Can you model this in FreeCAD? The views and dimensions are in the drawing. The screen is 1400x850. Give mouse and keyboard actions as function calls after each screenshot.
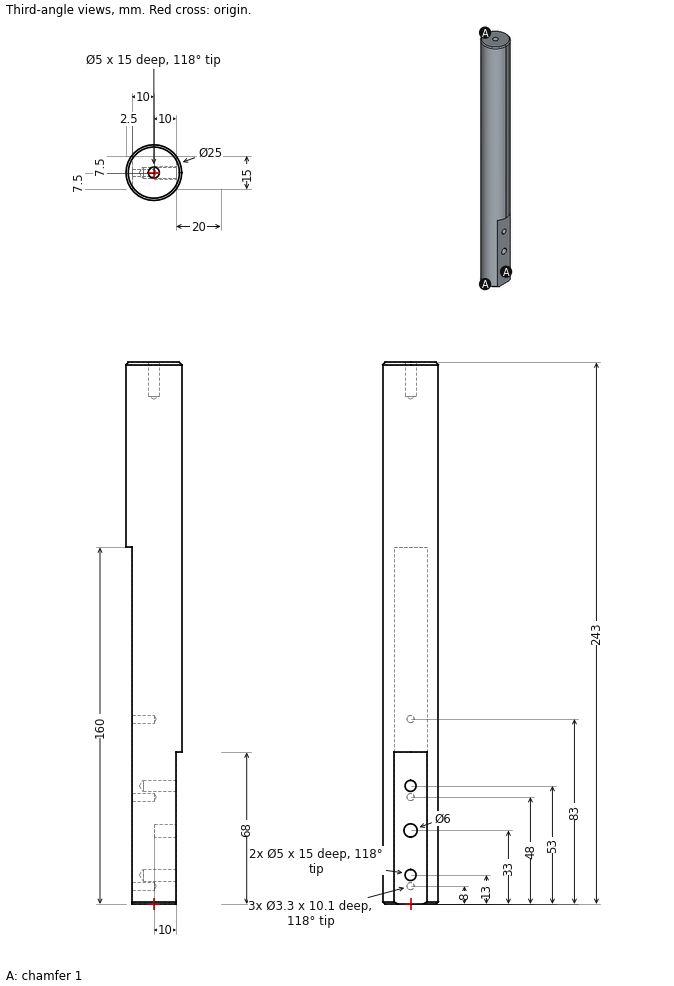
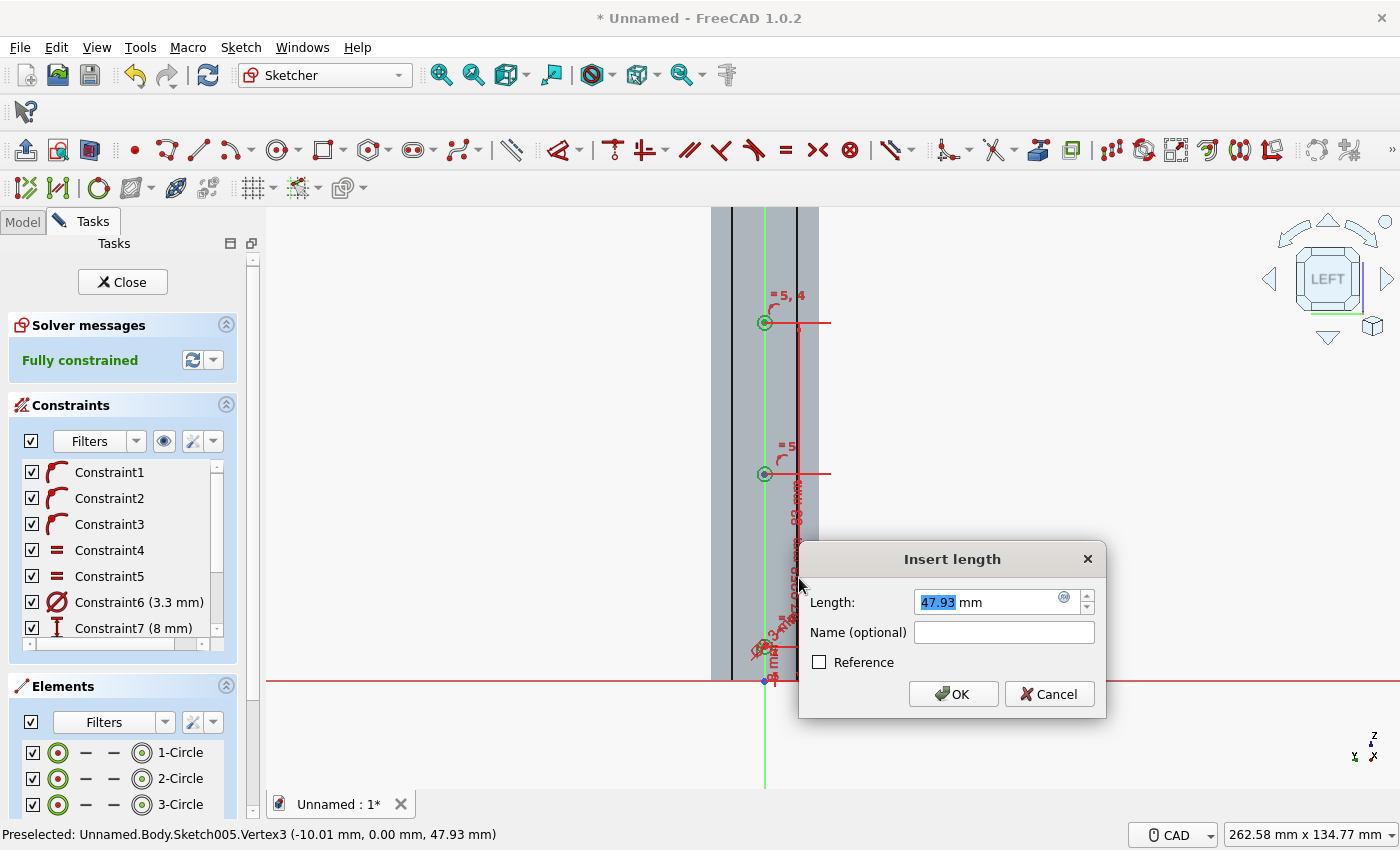
text(48)
key(Return)
key(Escape)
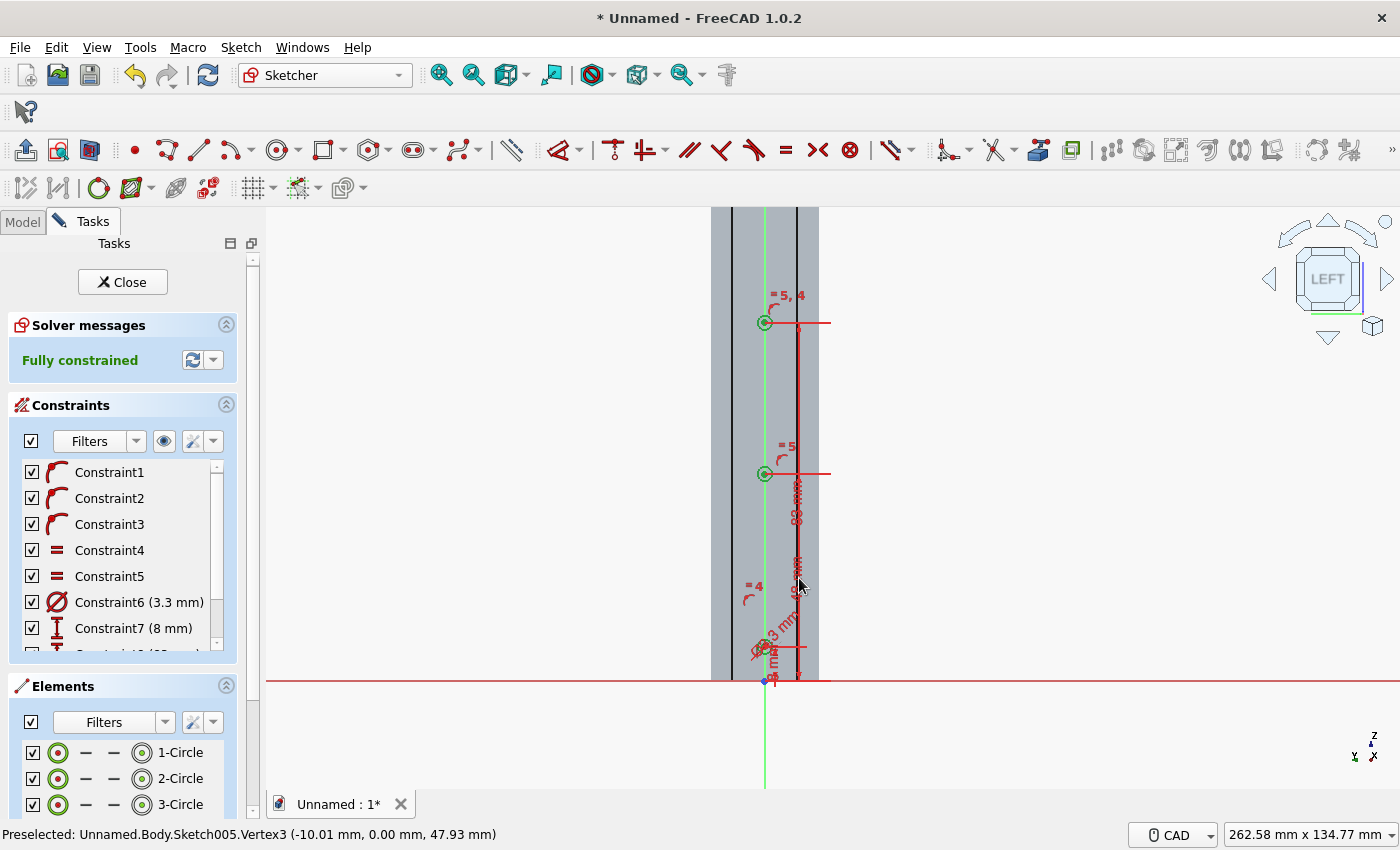
click(123, 282)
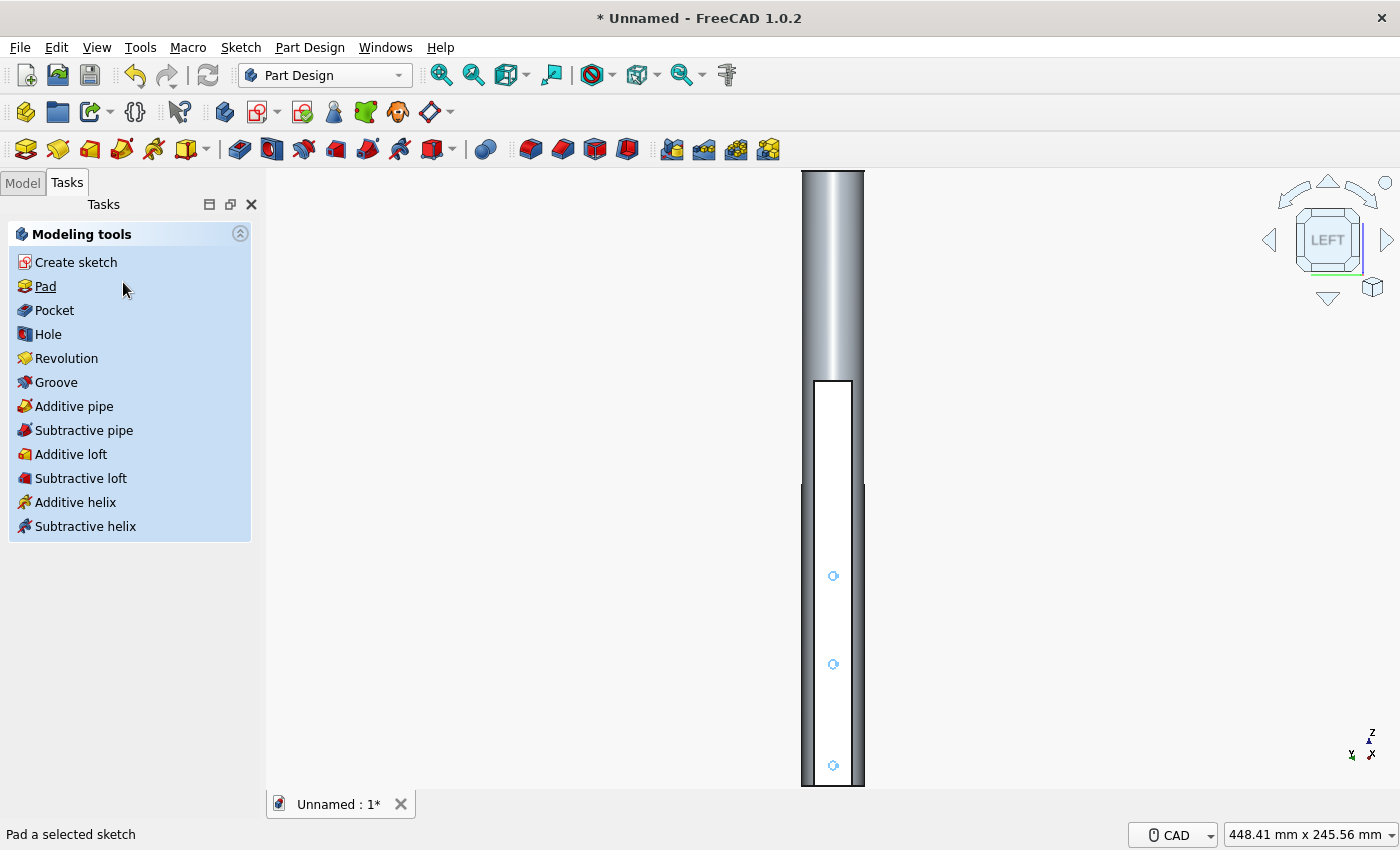
click(272, 150)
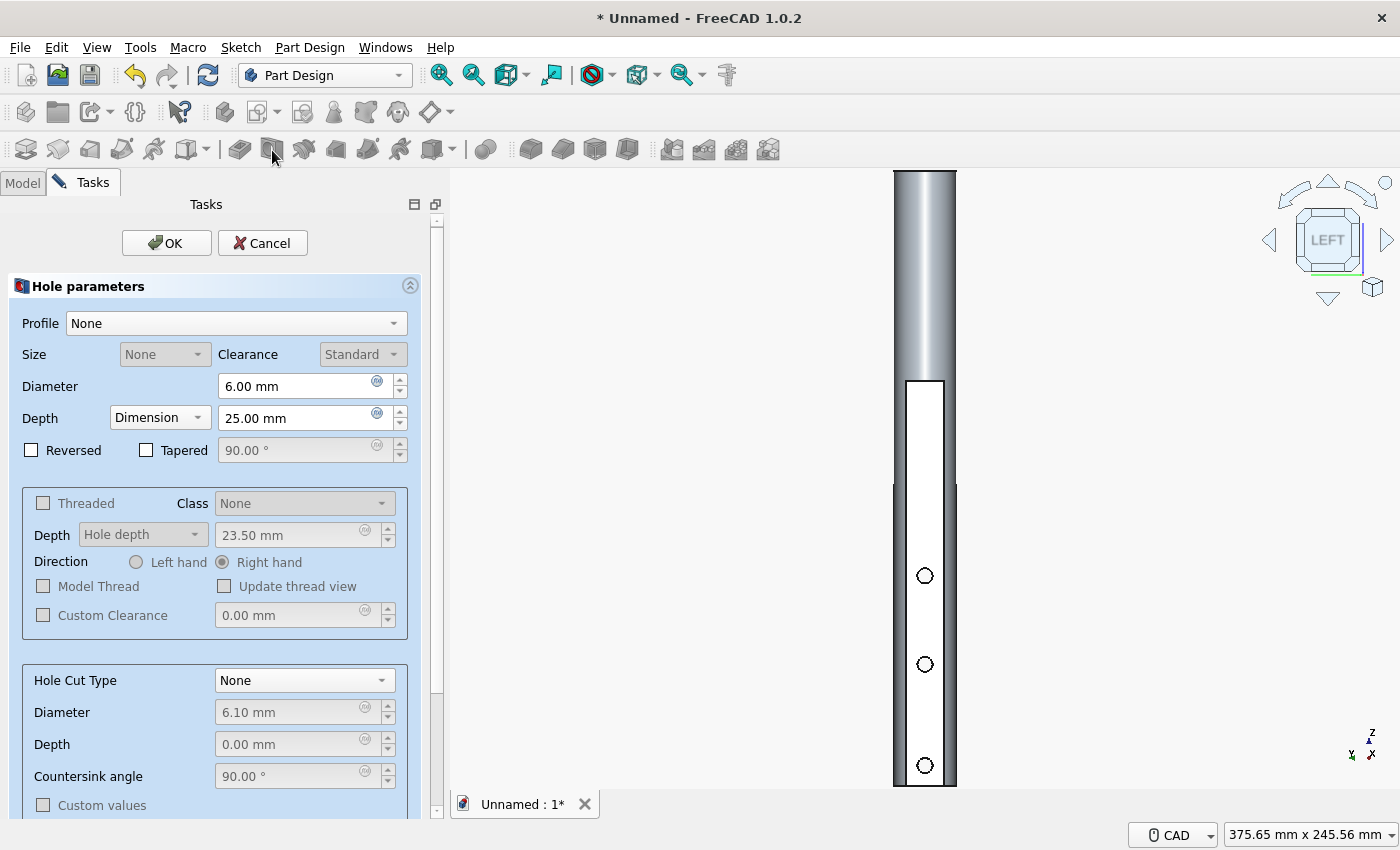
triple_click(305, 386)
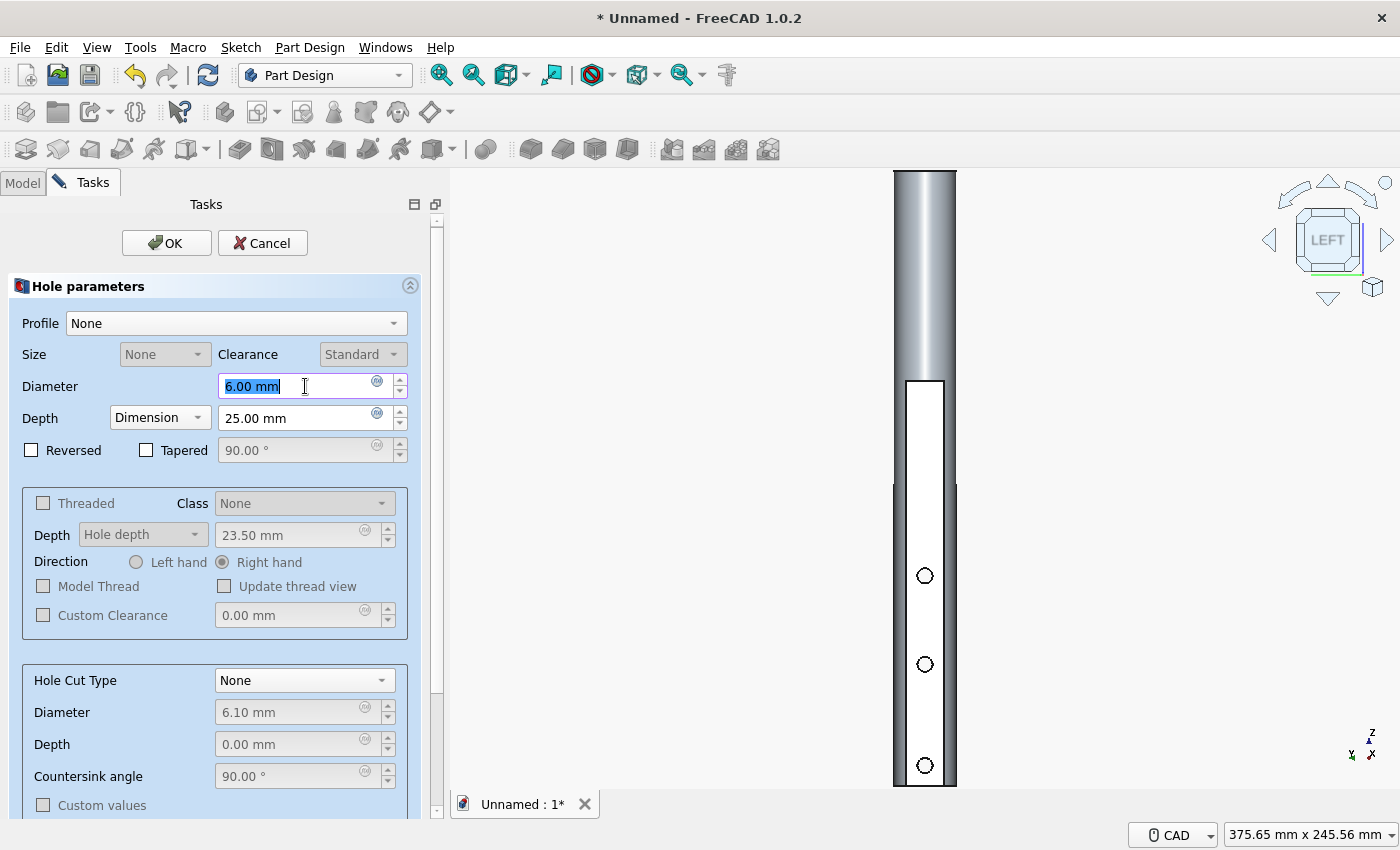
text(3.3)
key(Tab)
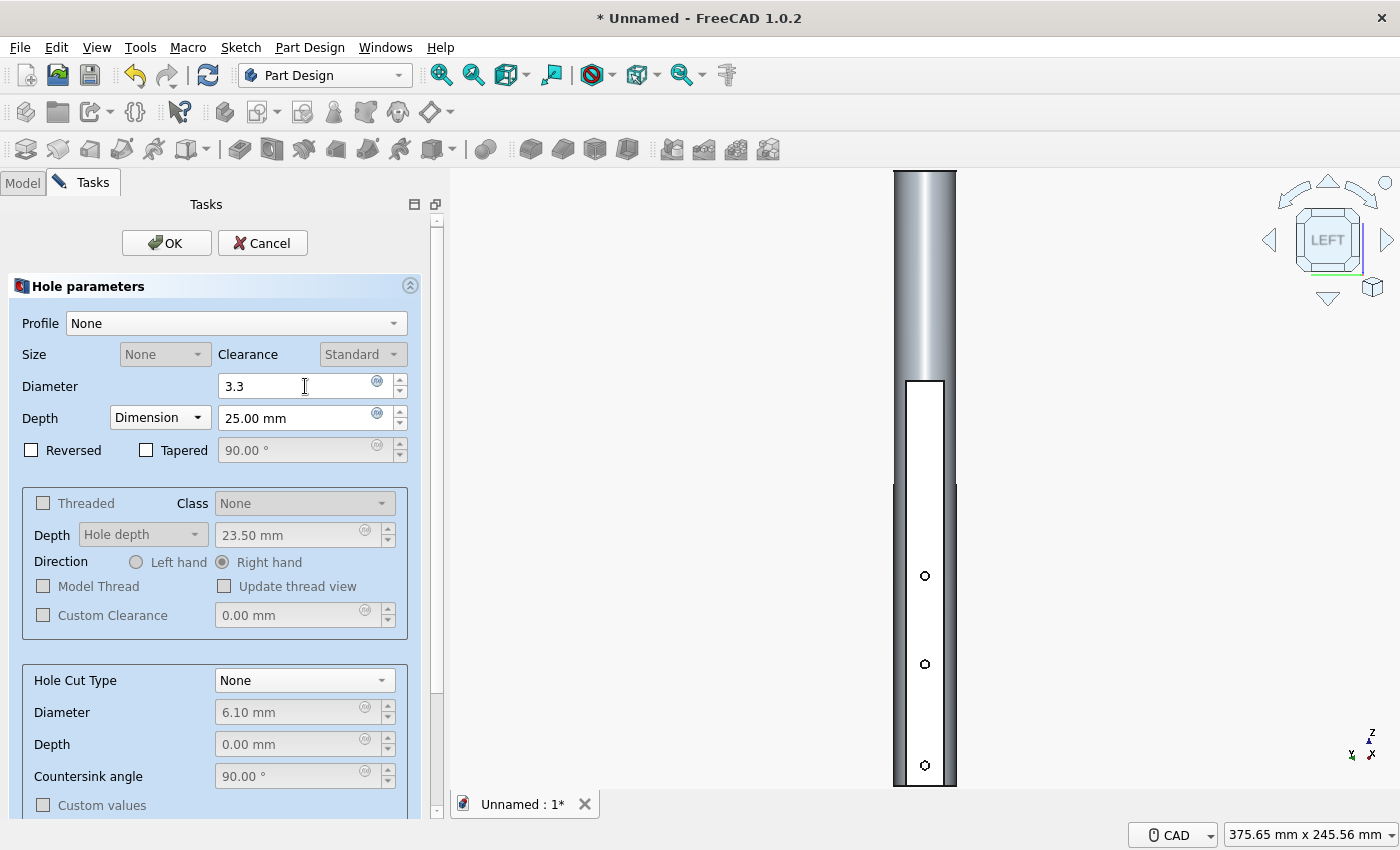
triple_click(305, 418)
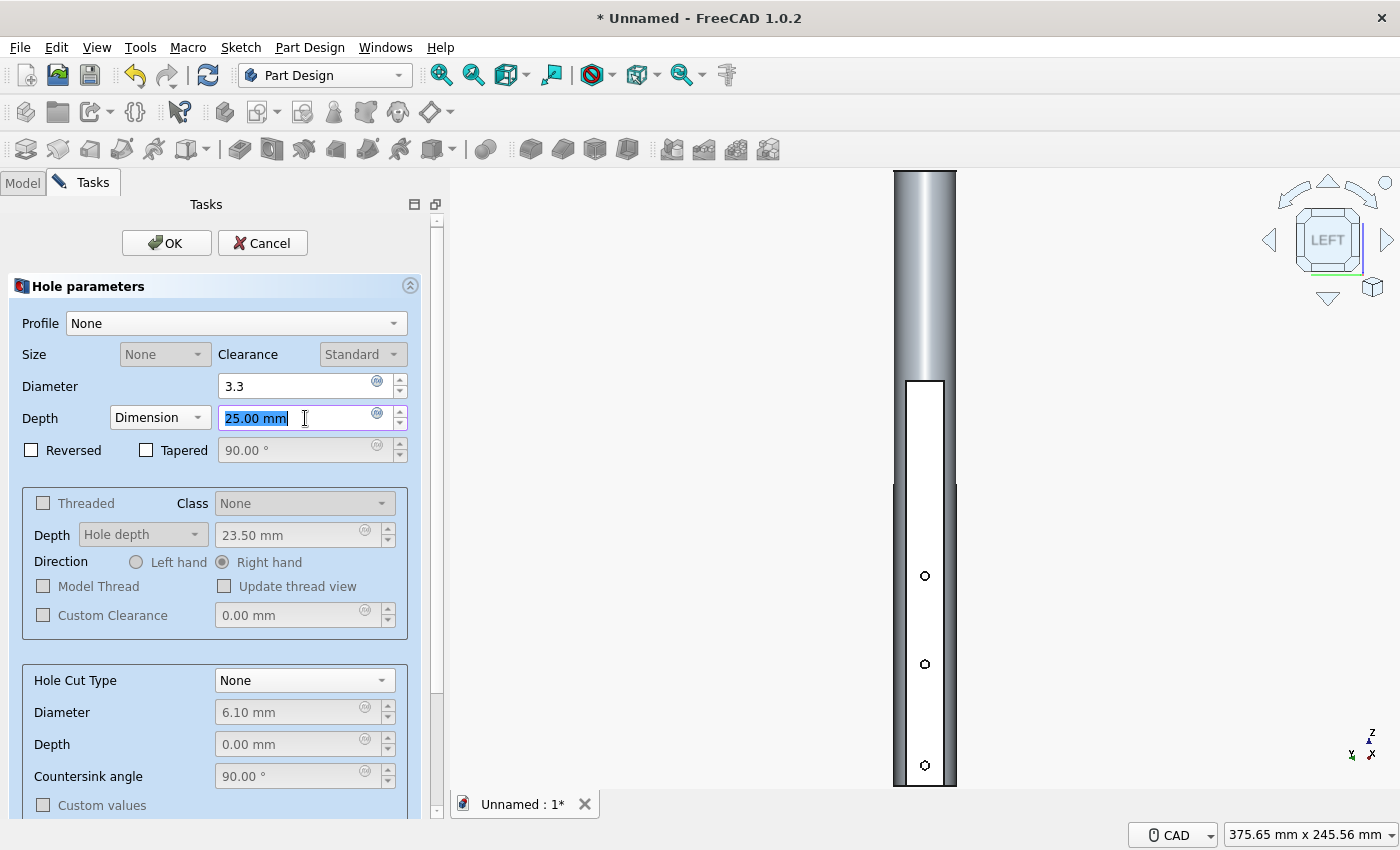
text(10.1)
key(Tab)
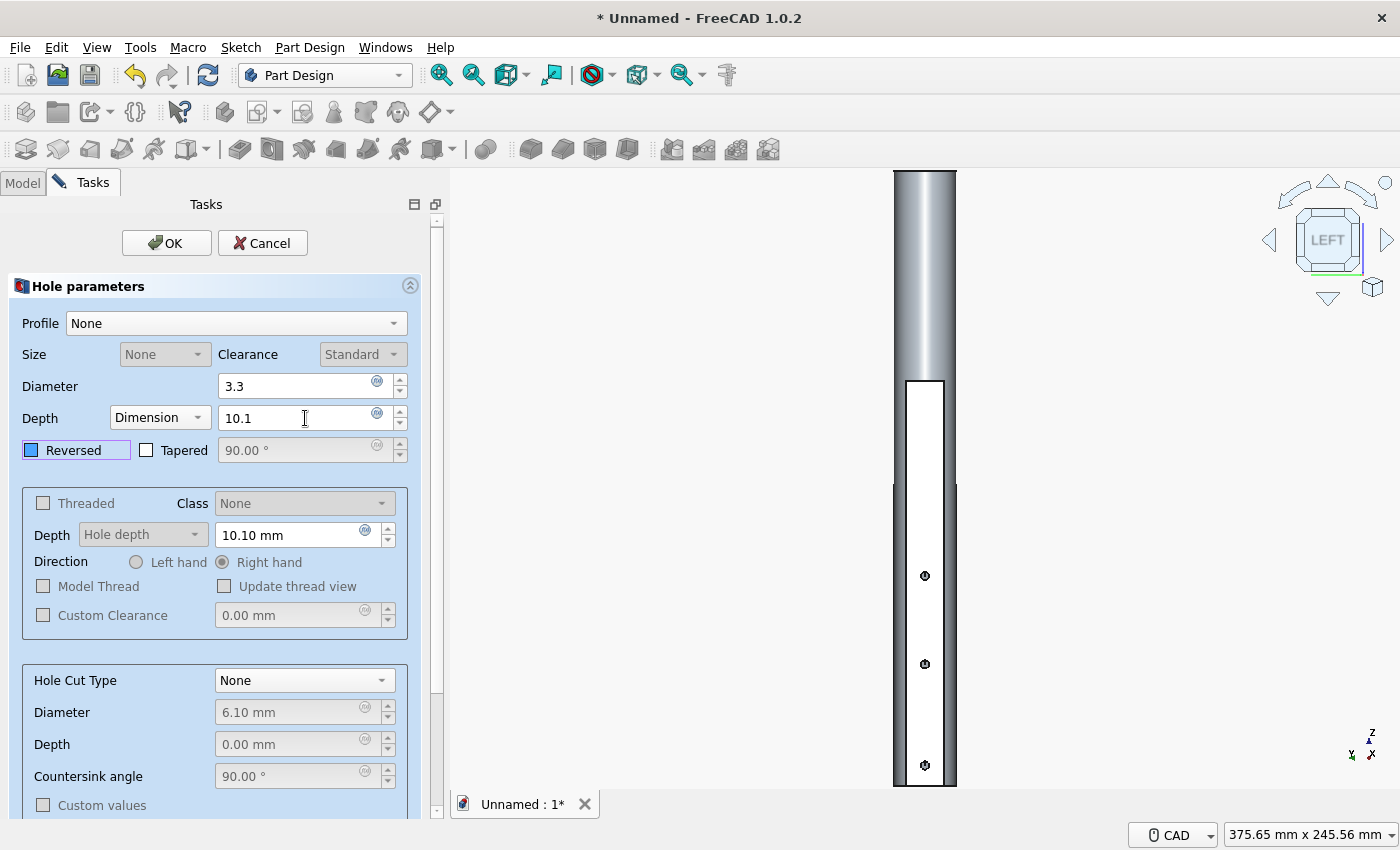
click(167, 243)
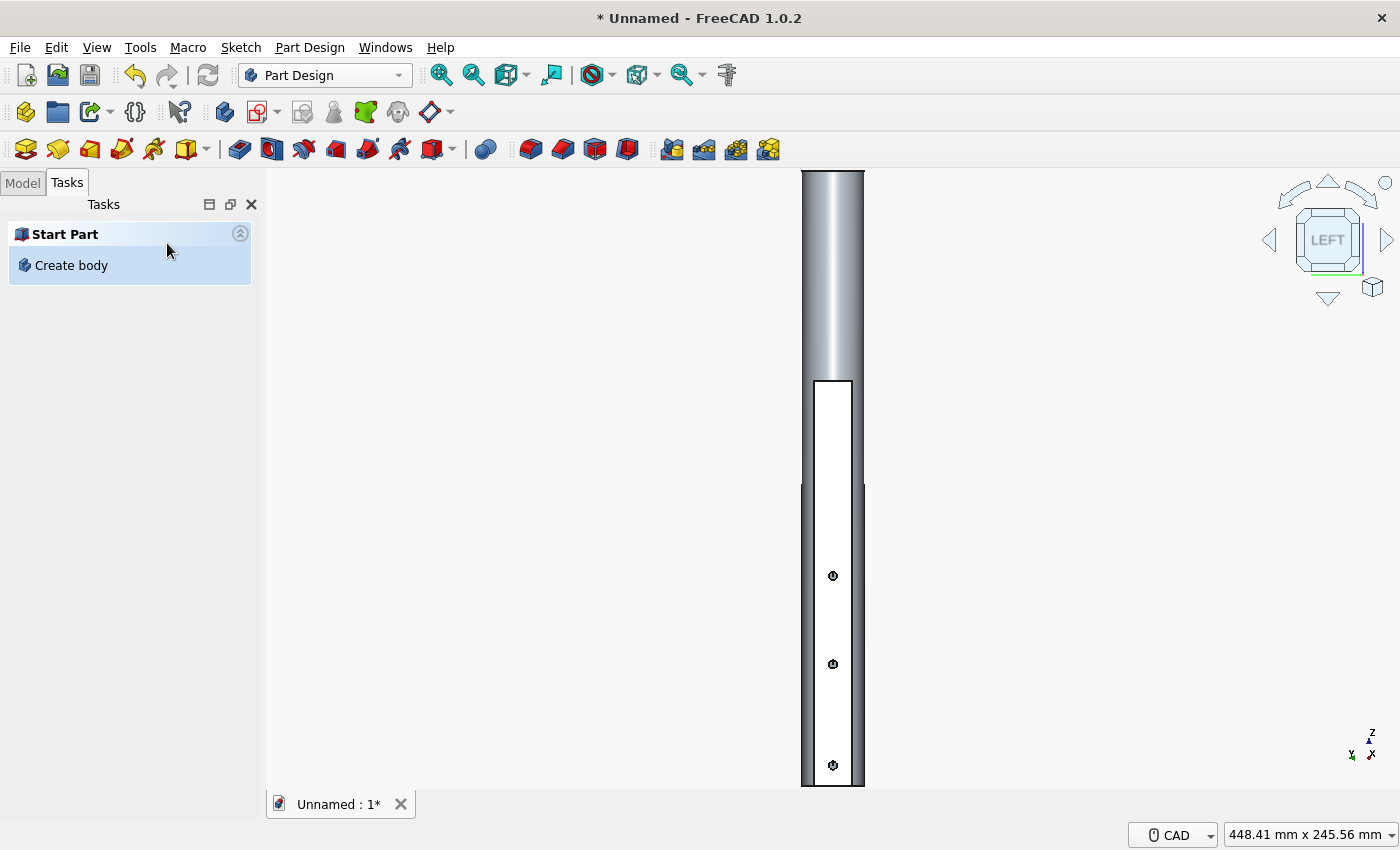
key(0)